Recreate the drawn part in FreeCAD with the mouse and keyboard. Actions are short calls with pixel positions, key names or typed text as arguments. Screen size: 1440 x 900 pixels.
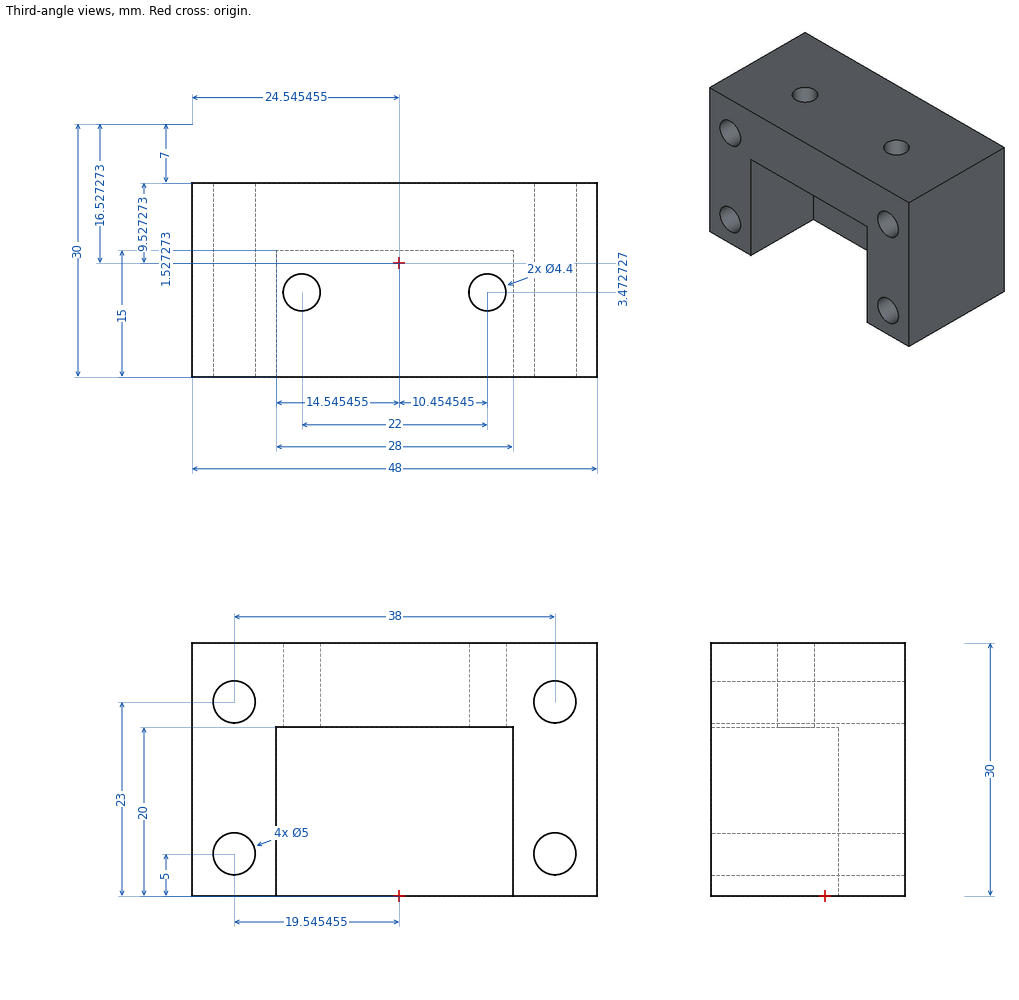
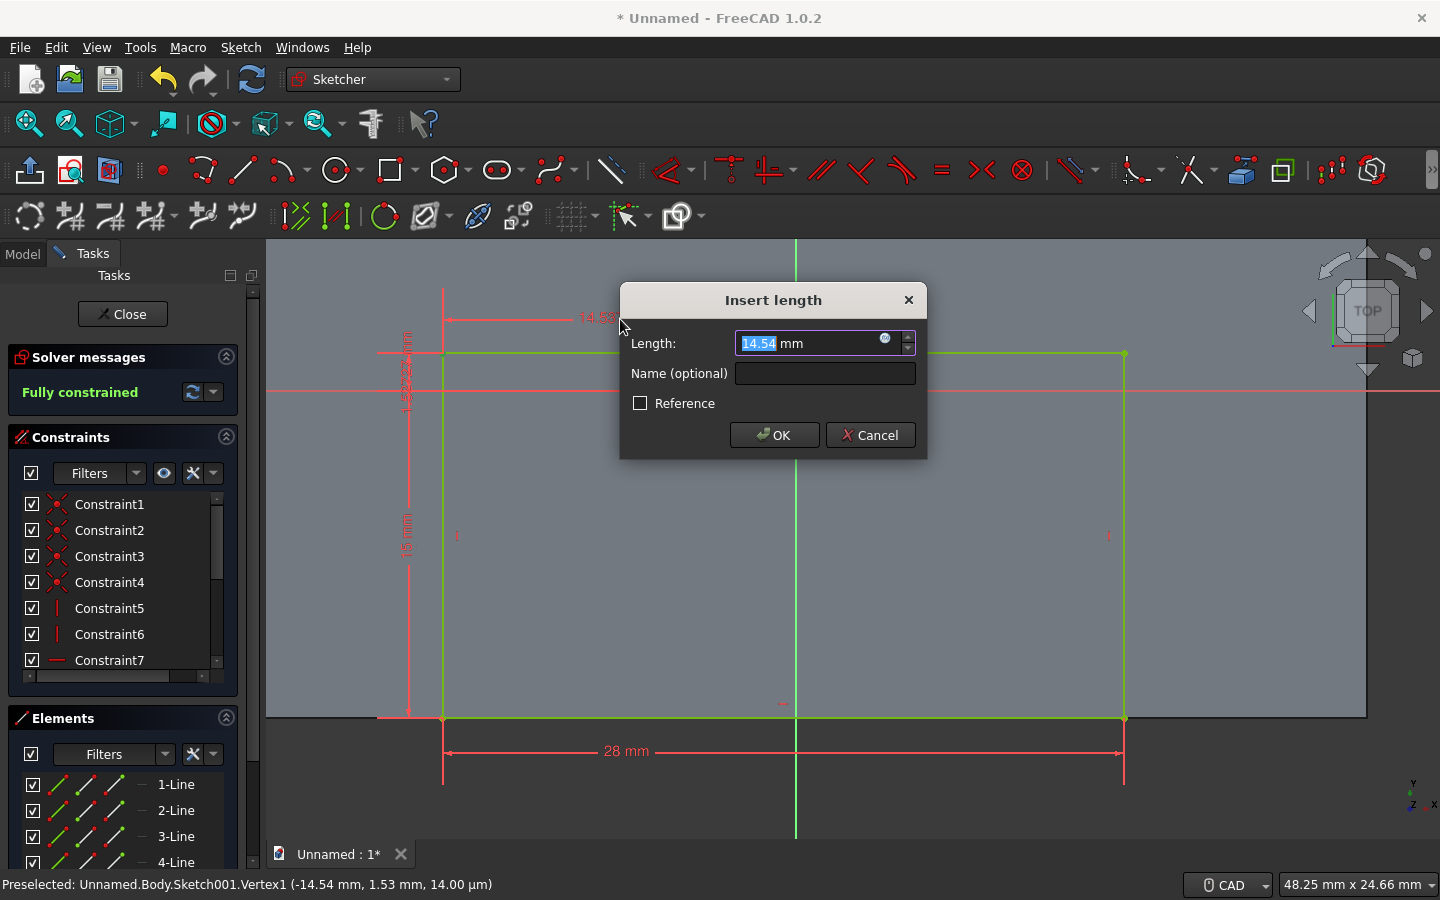
text(14.545455)
key(Return)
key(Escape)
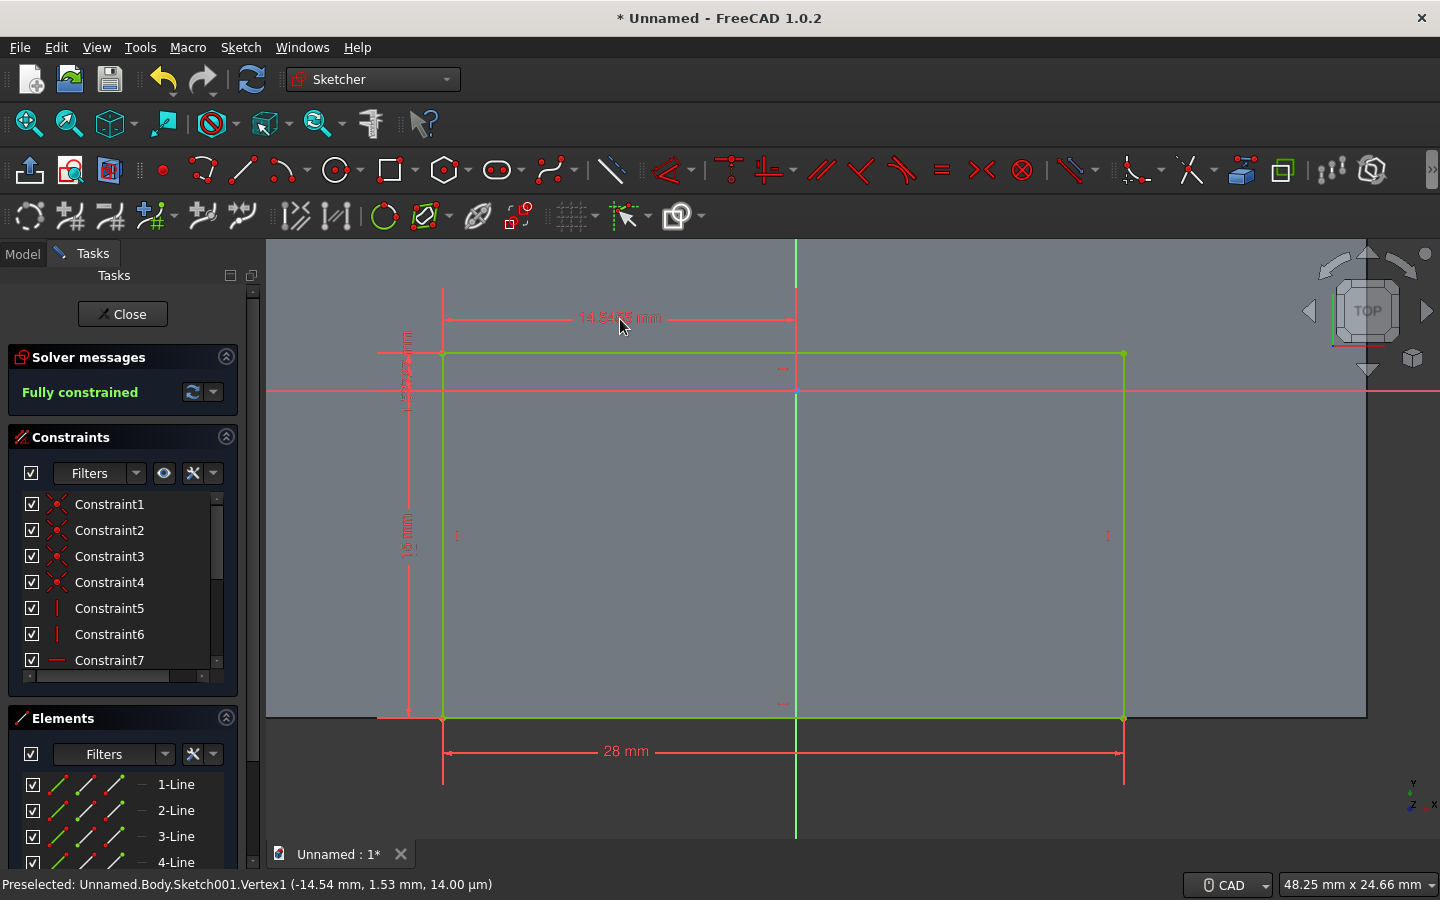
click(123, 314)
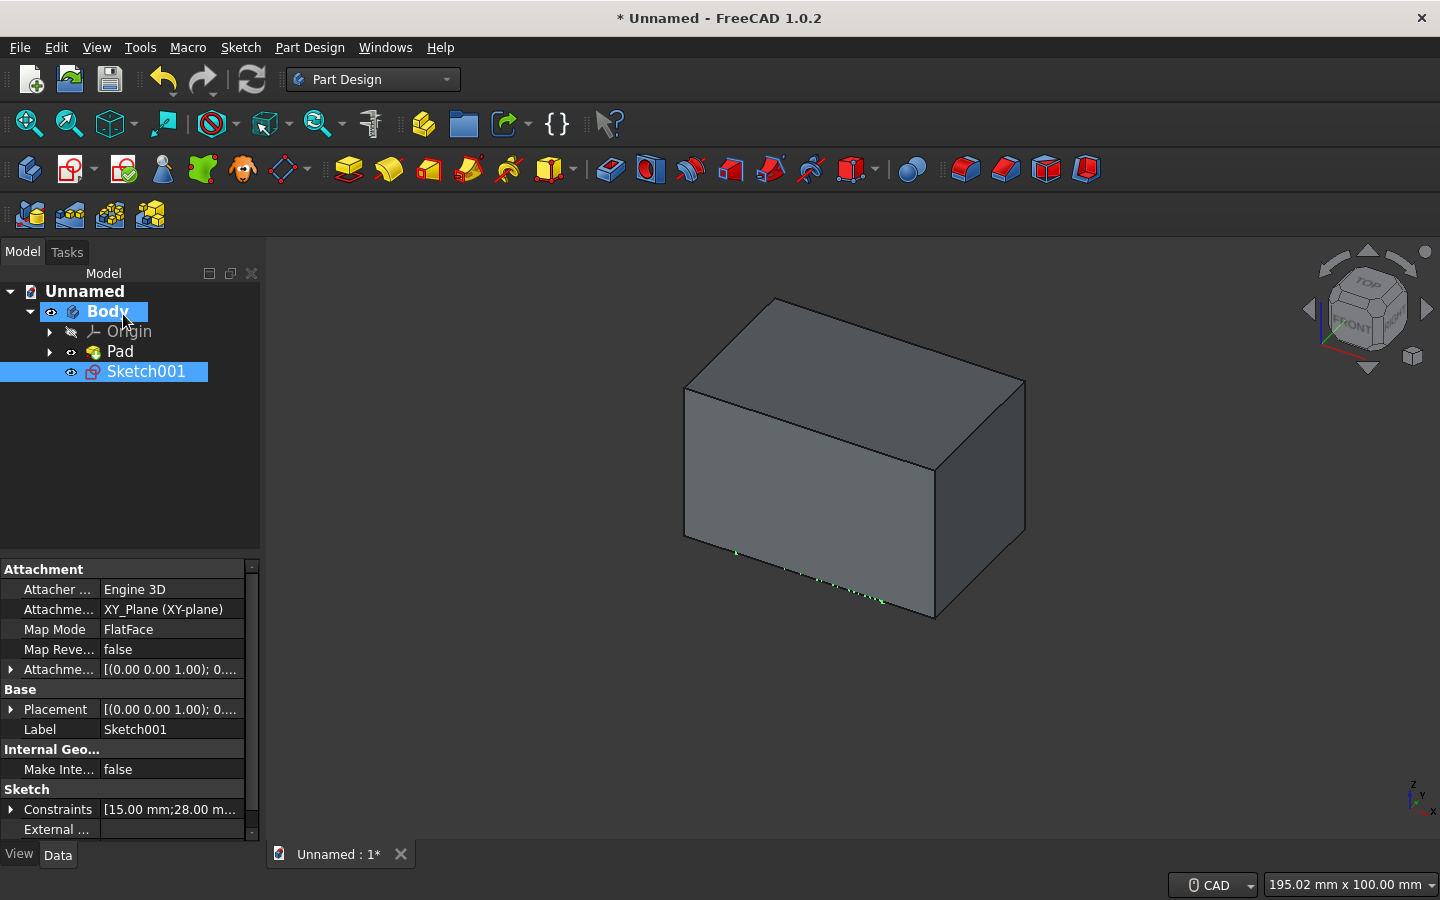
click(612, 170)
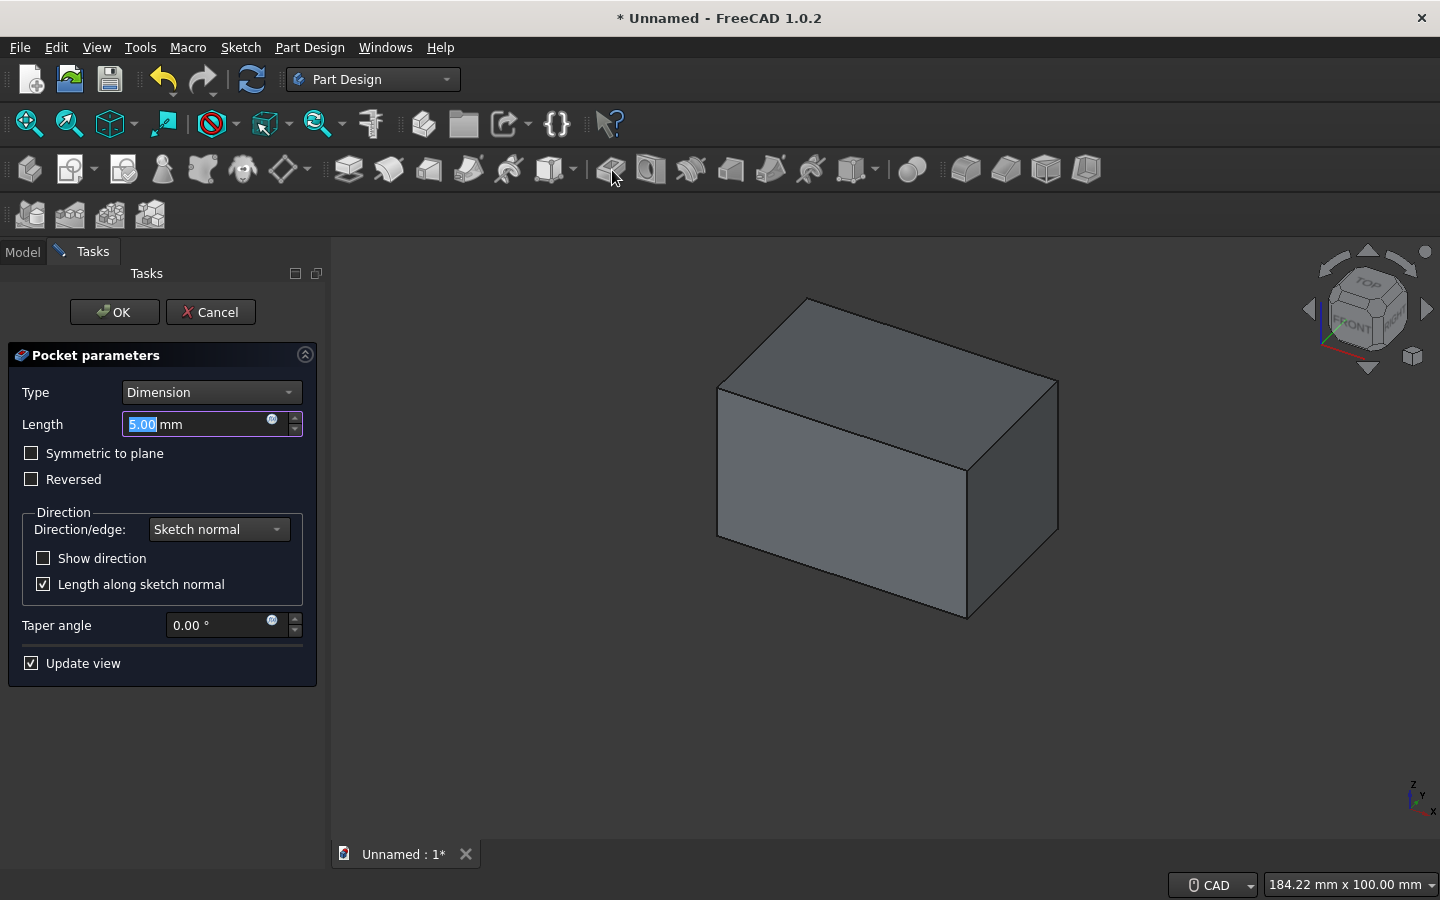
text(20)
key(Tab)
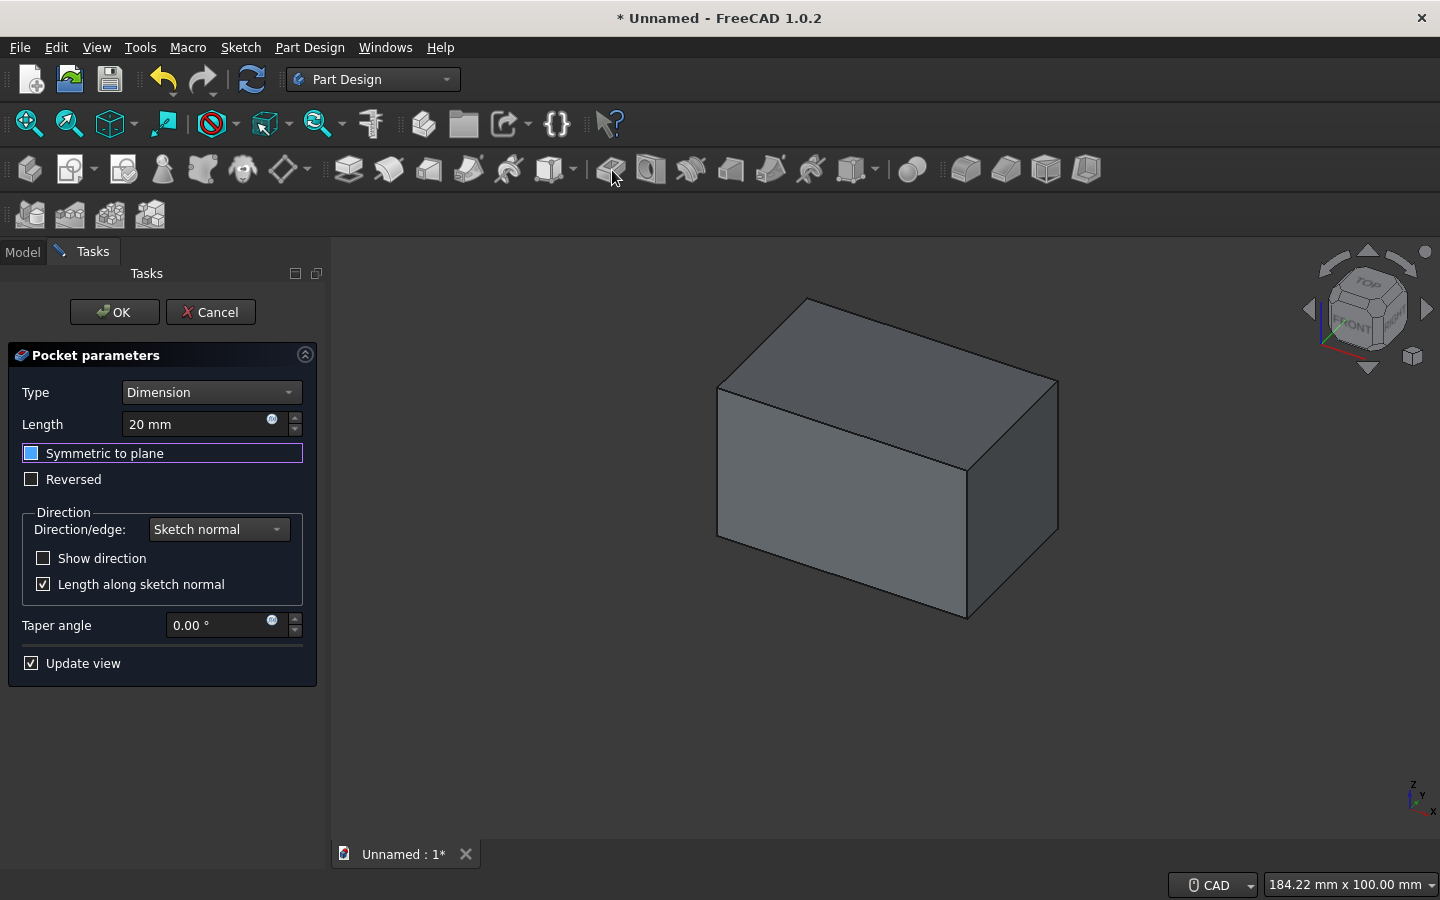
click(30, 479)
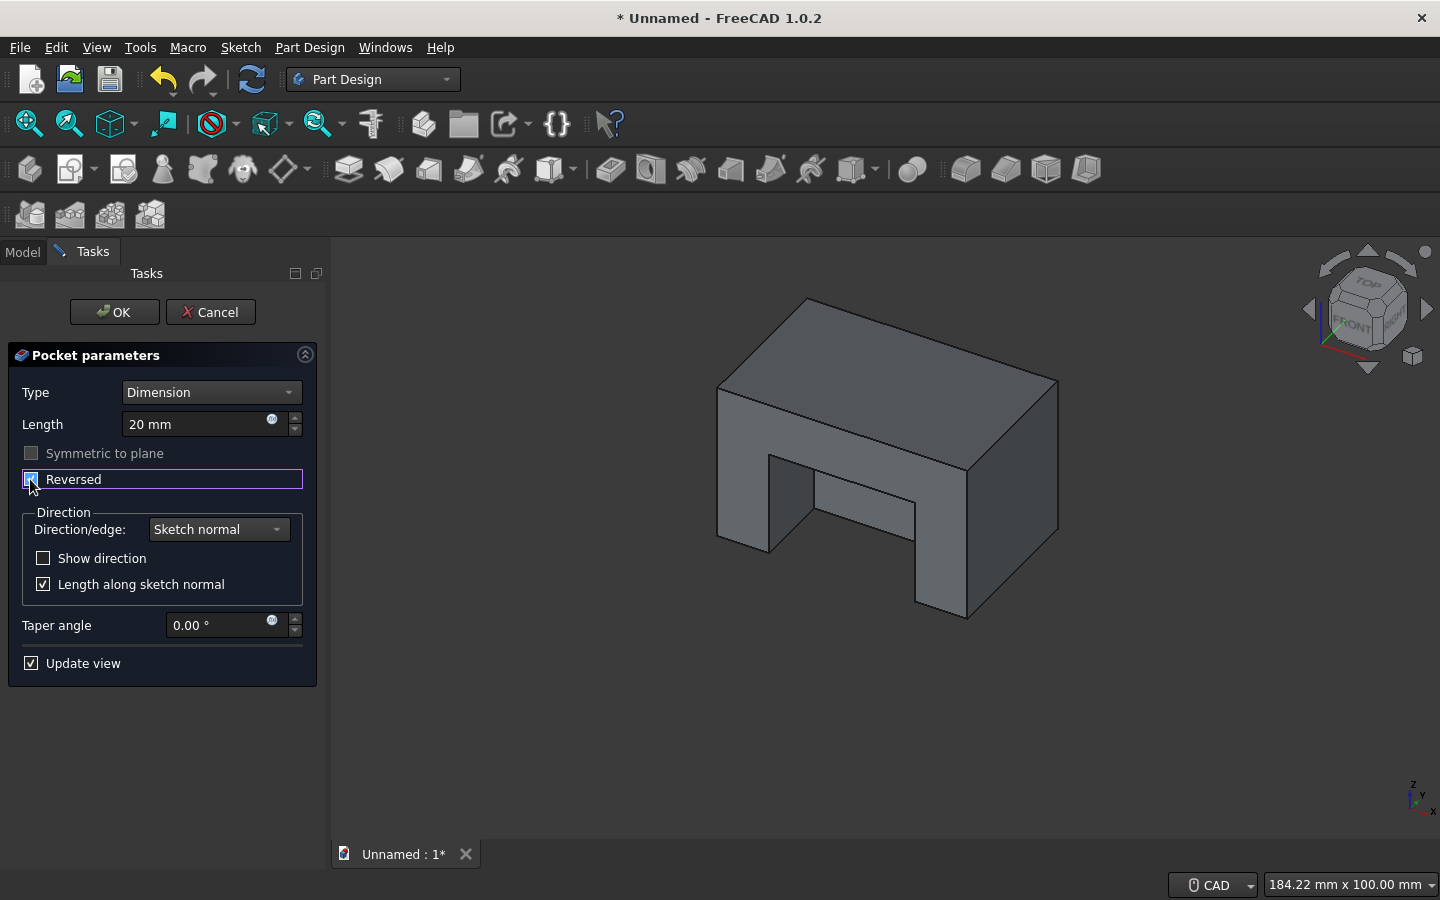
click(115, 312)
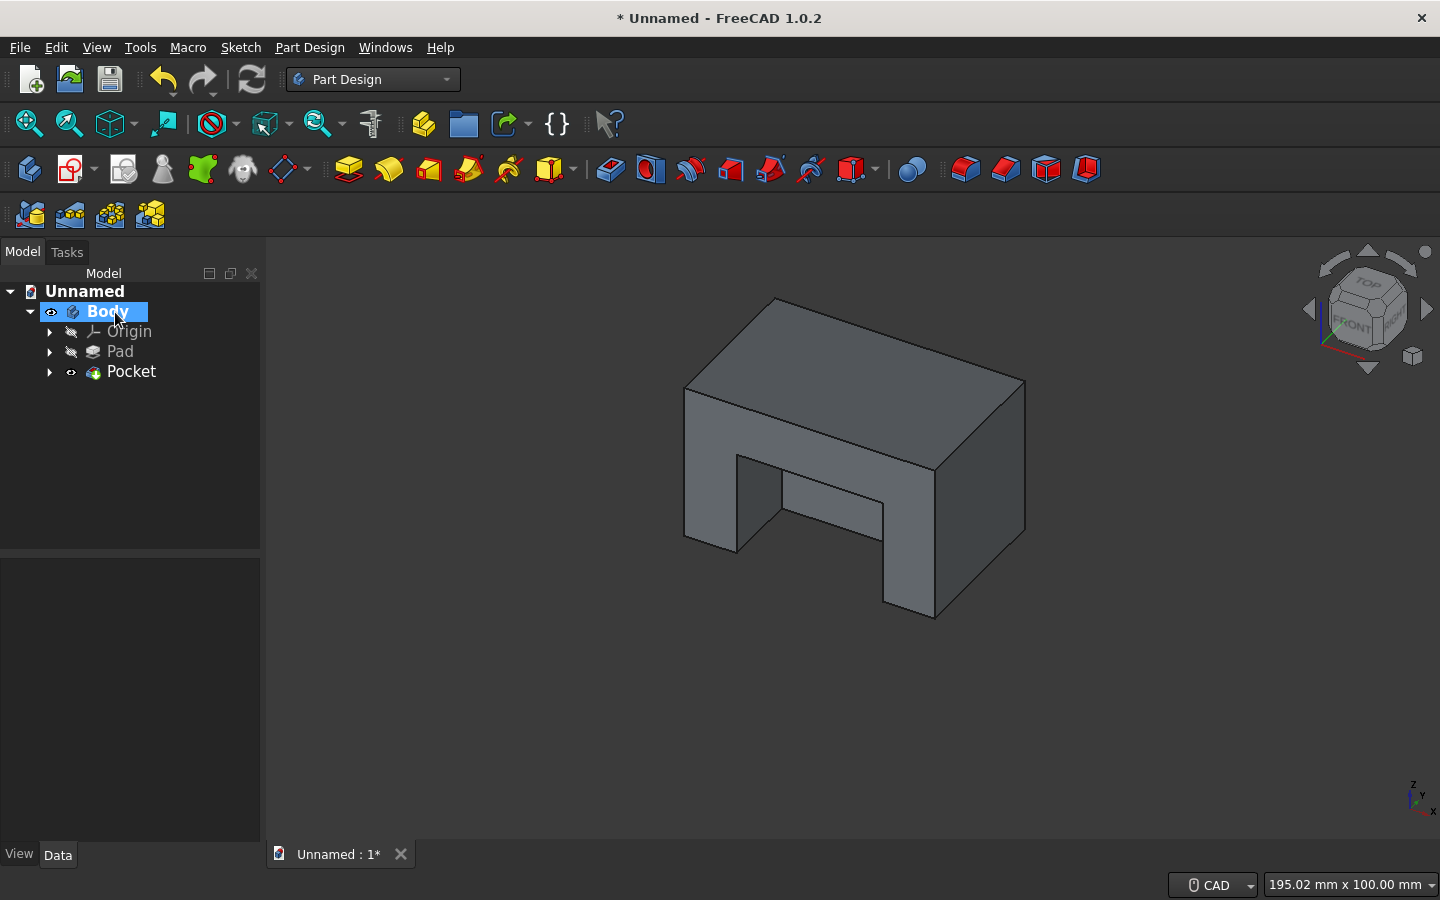
key(5)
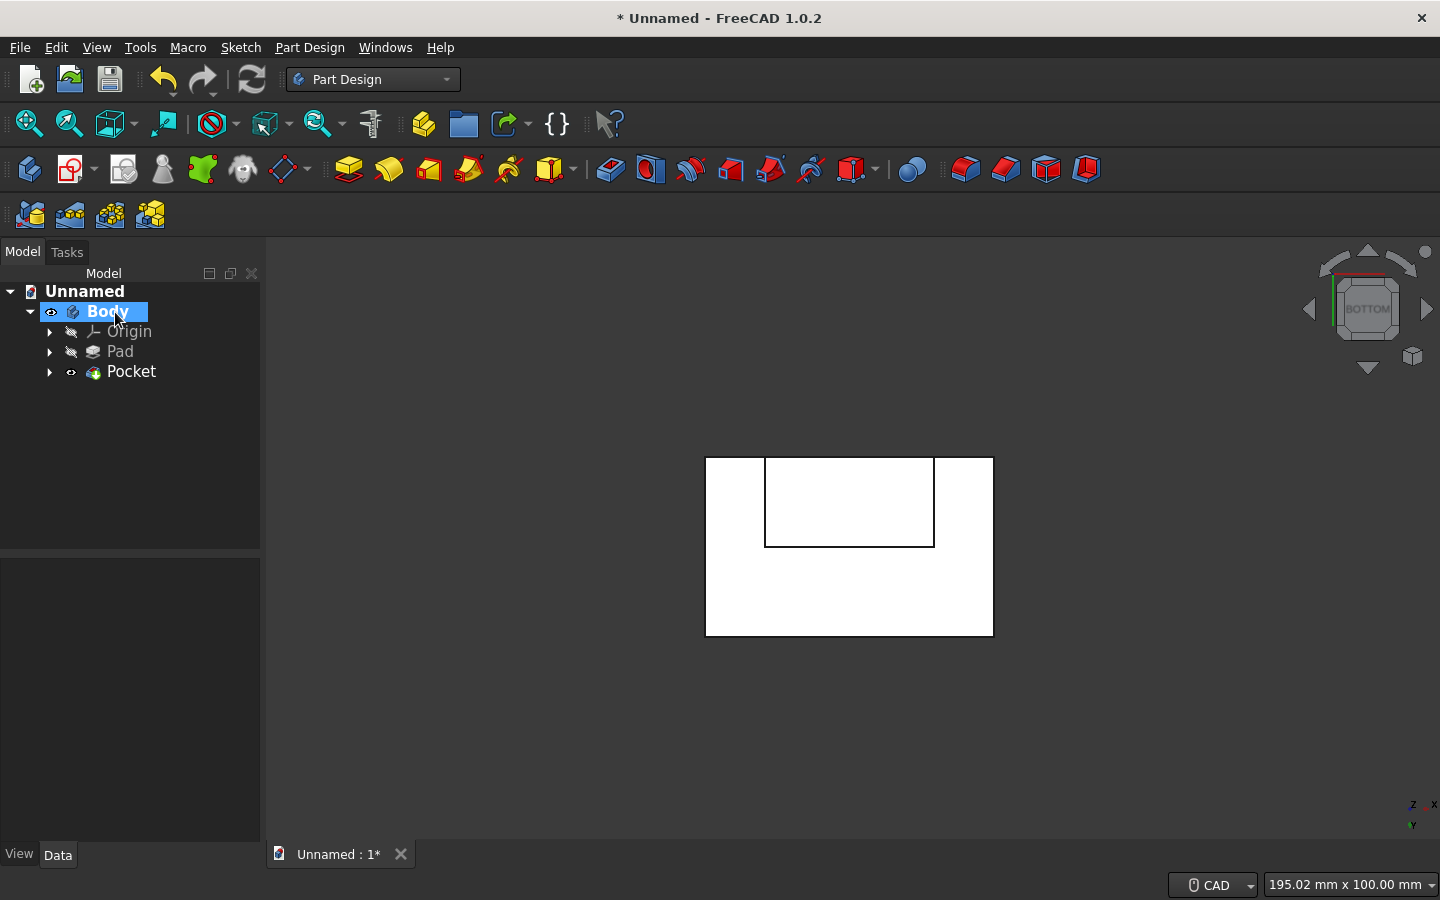
click(30, 124)